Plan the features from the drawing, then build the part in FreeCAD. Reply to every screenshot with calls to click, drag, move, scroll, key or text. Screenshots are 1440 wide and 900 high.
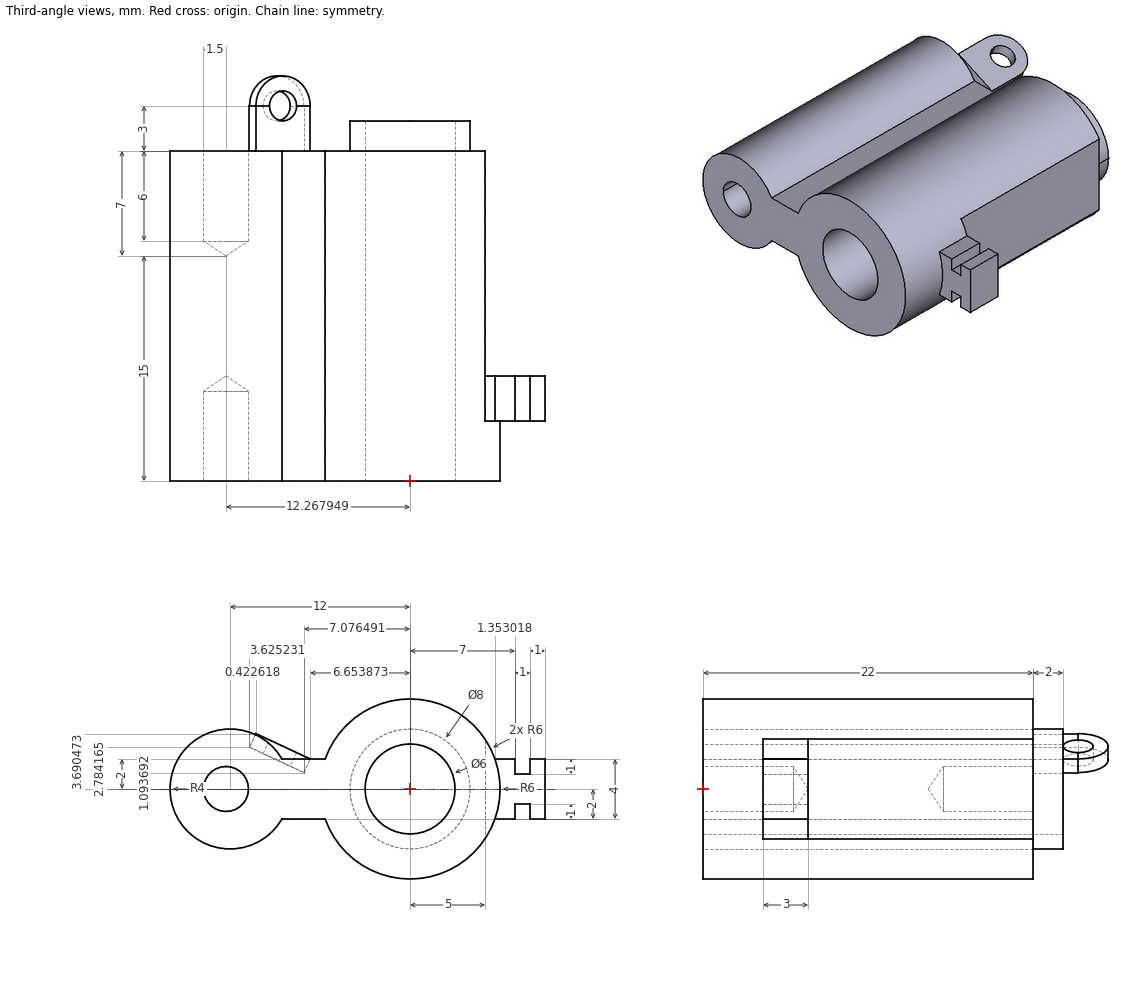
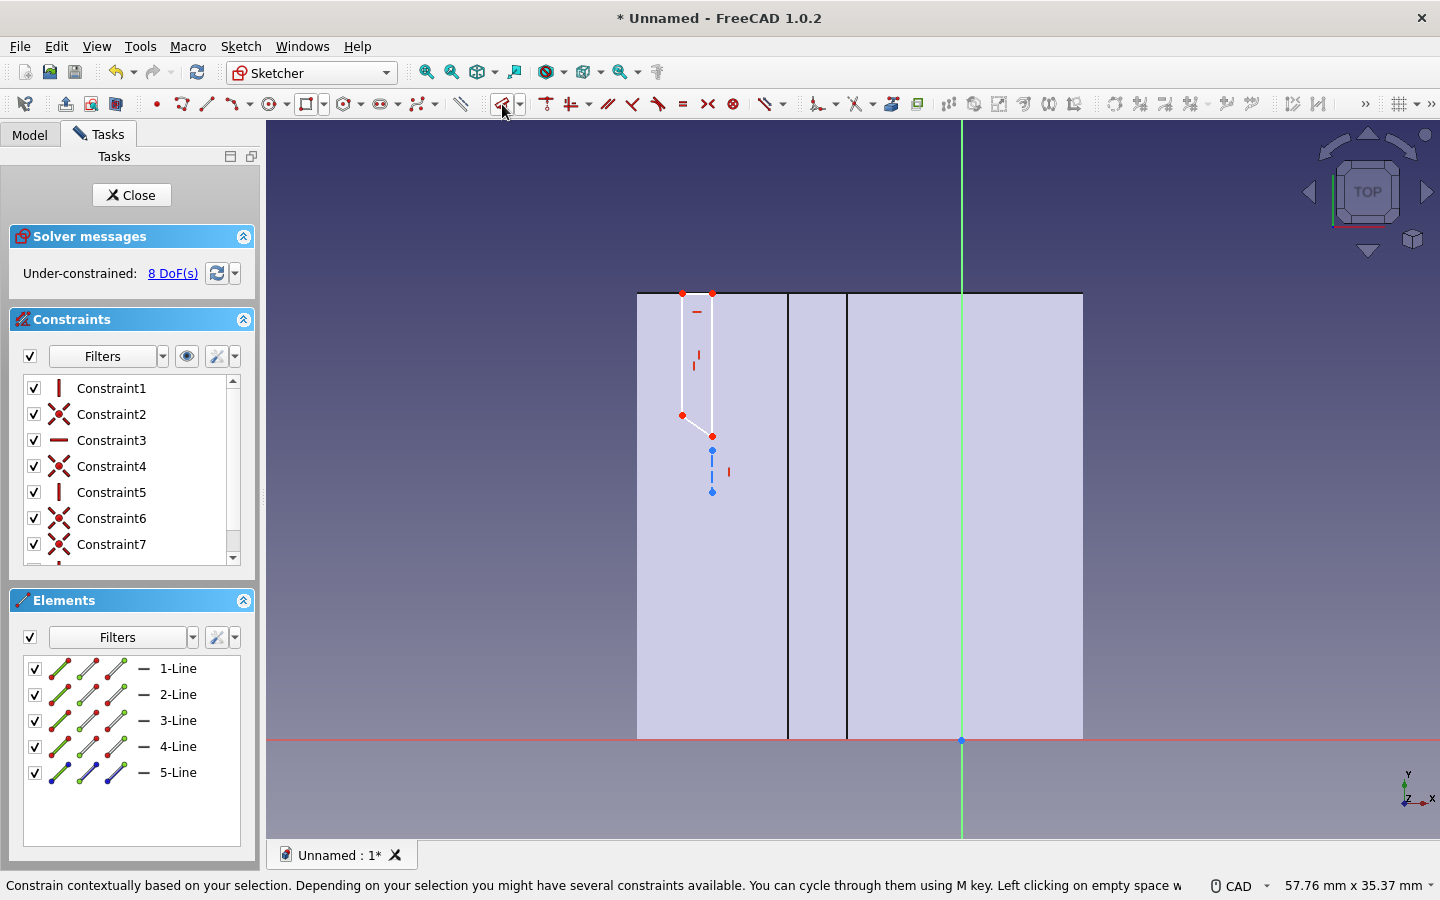
click(712, 394)
click(746, 366)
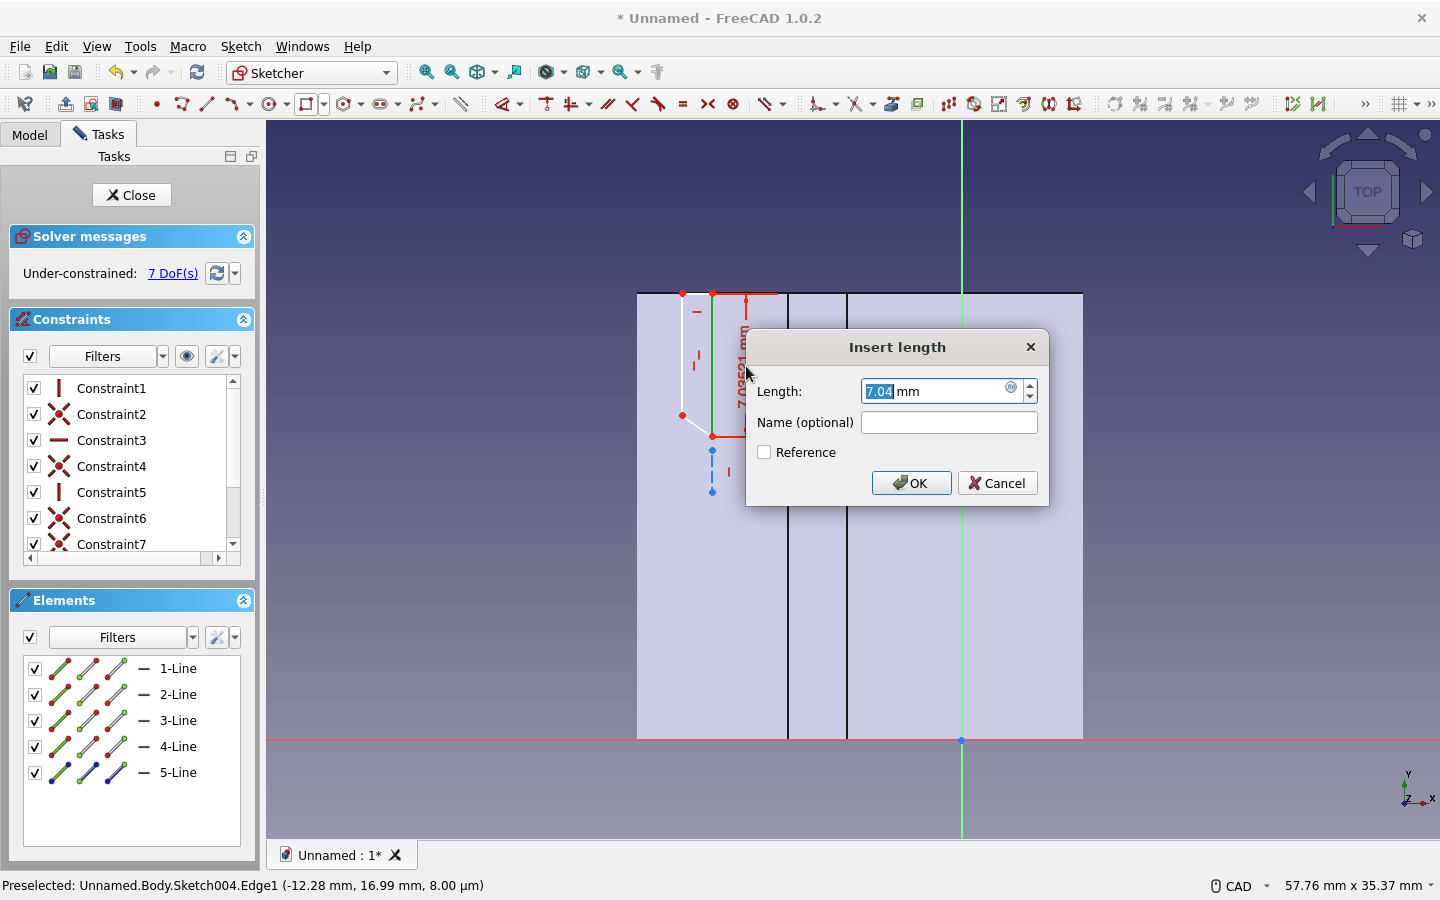
text(7)
key(Return)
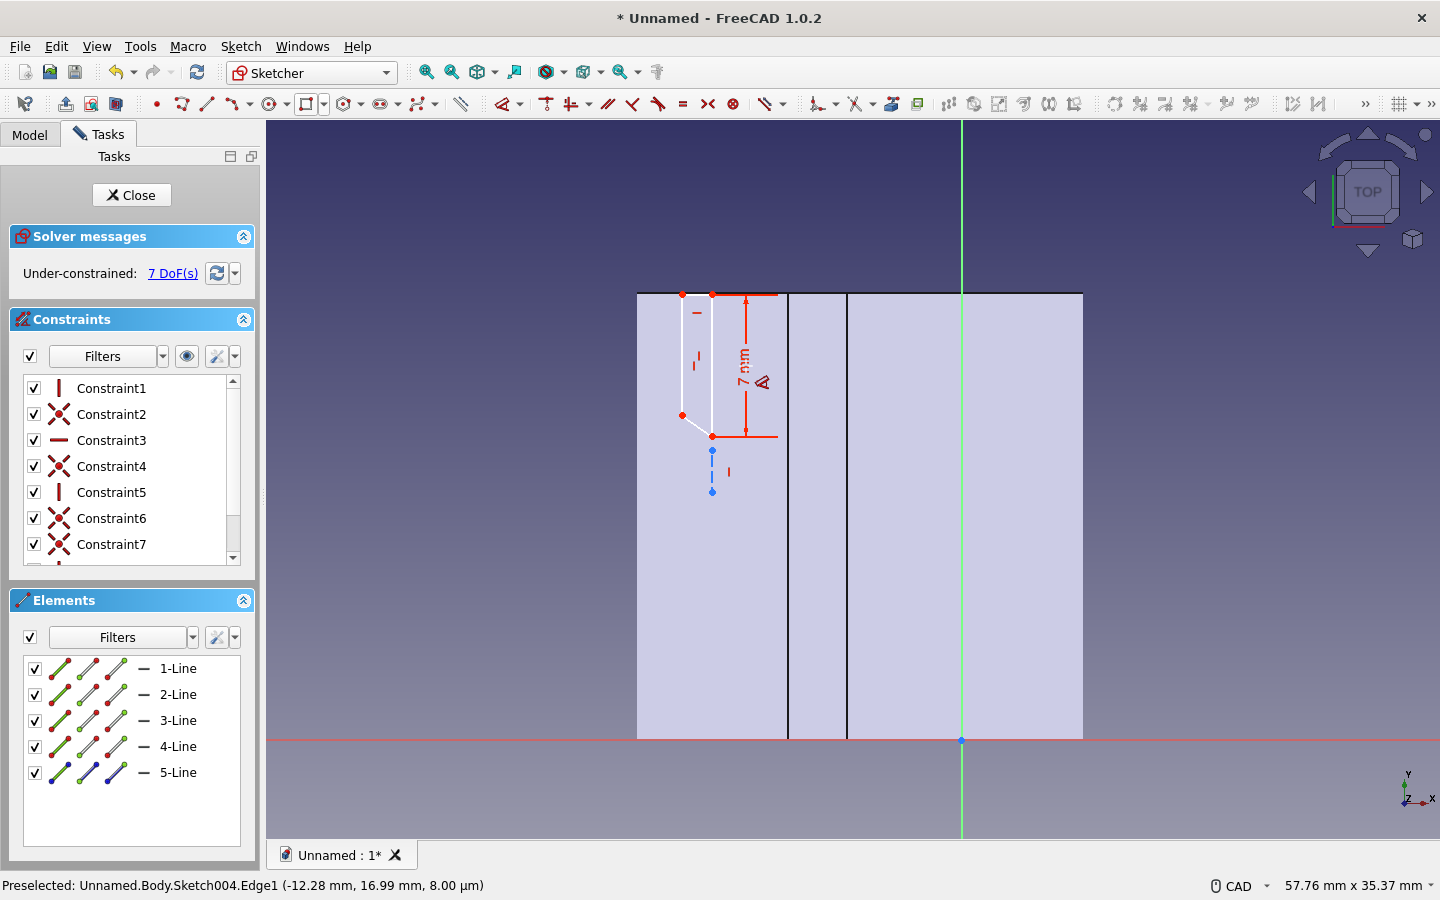
click(682, 331)
click(648, 355)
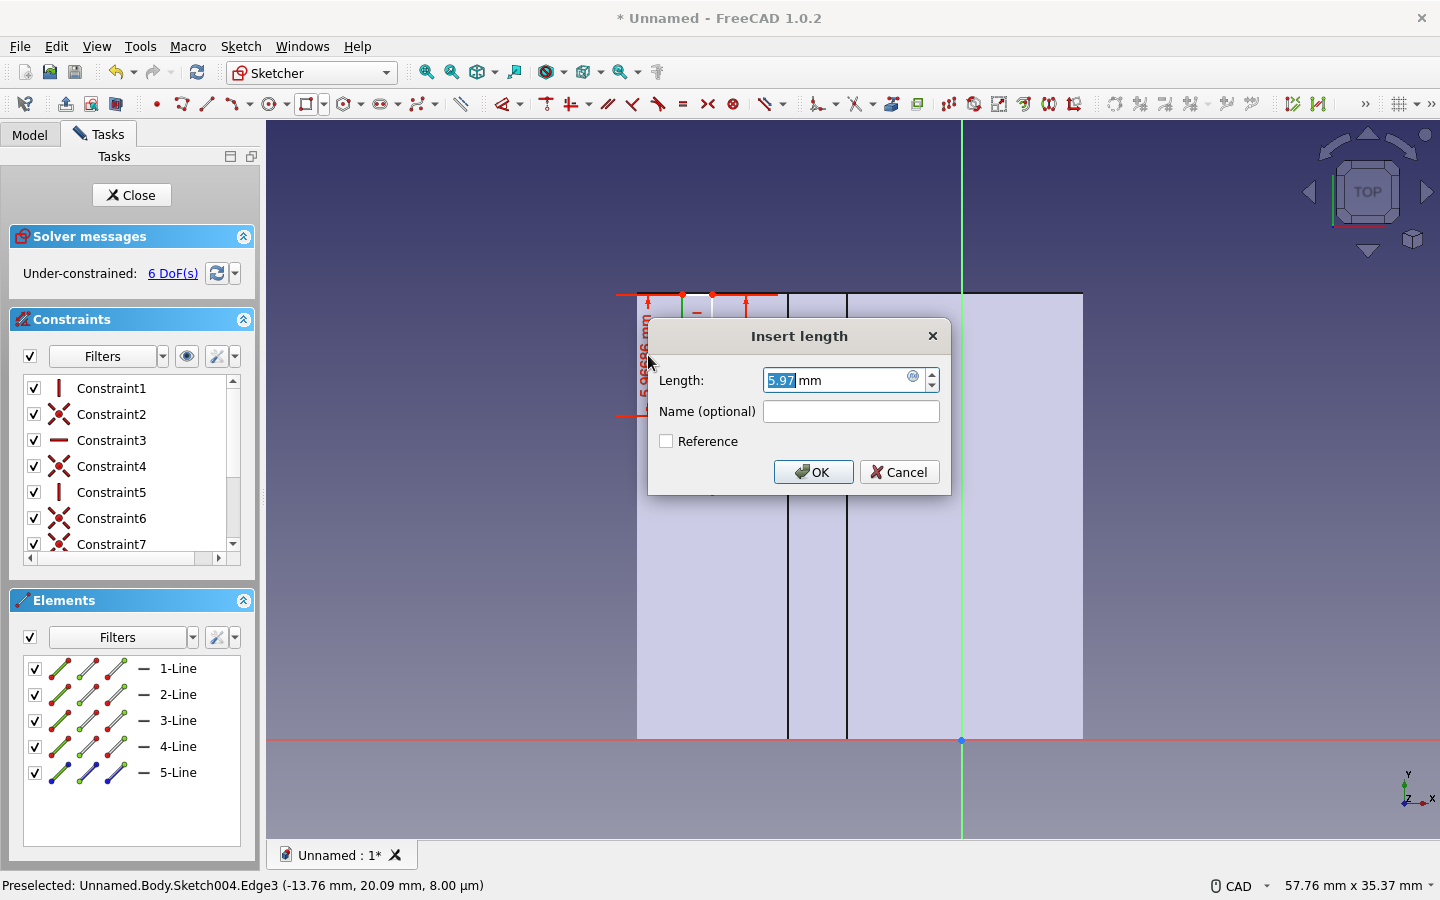
text(6)
key(Return)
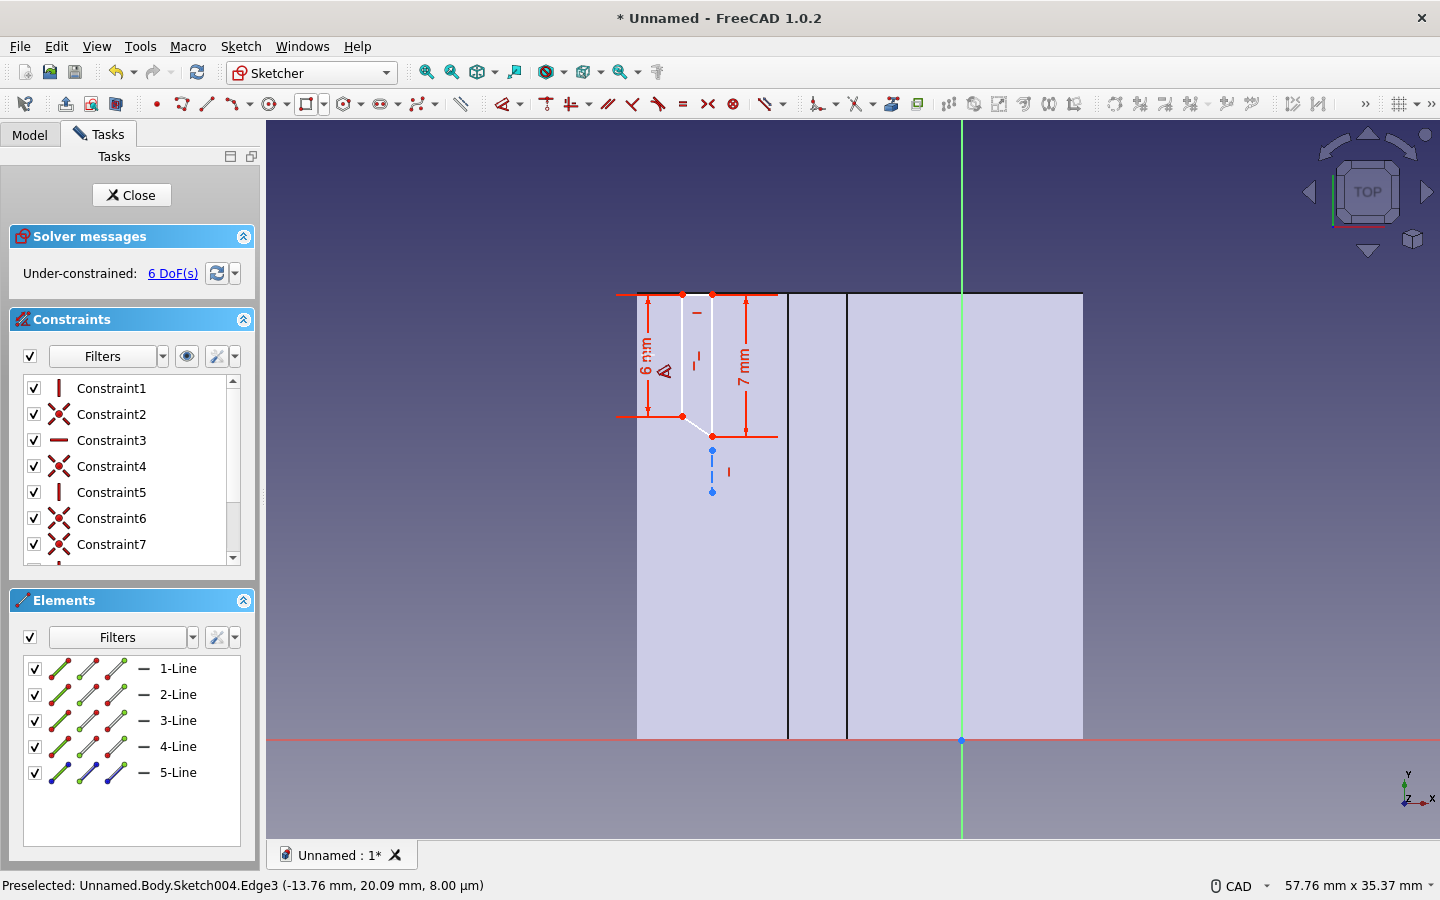
scroll(700, 295, up, 2)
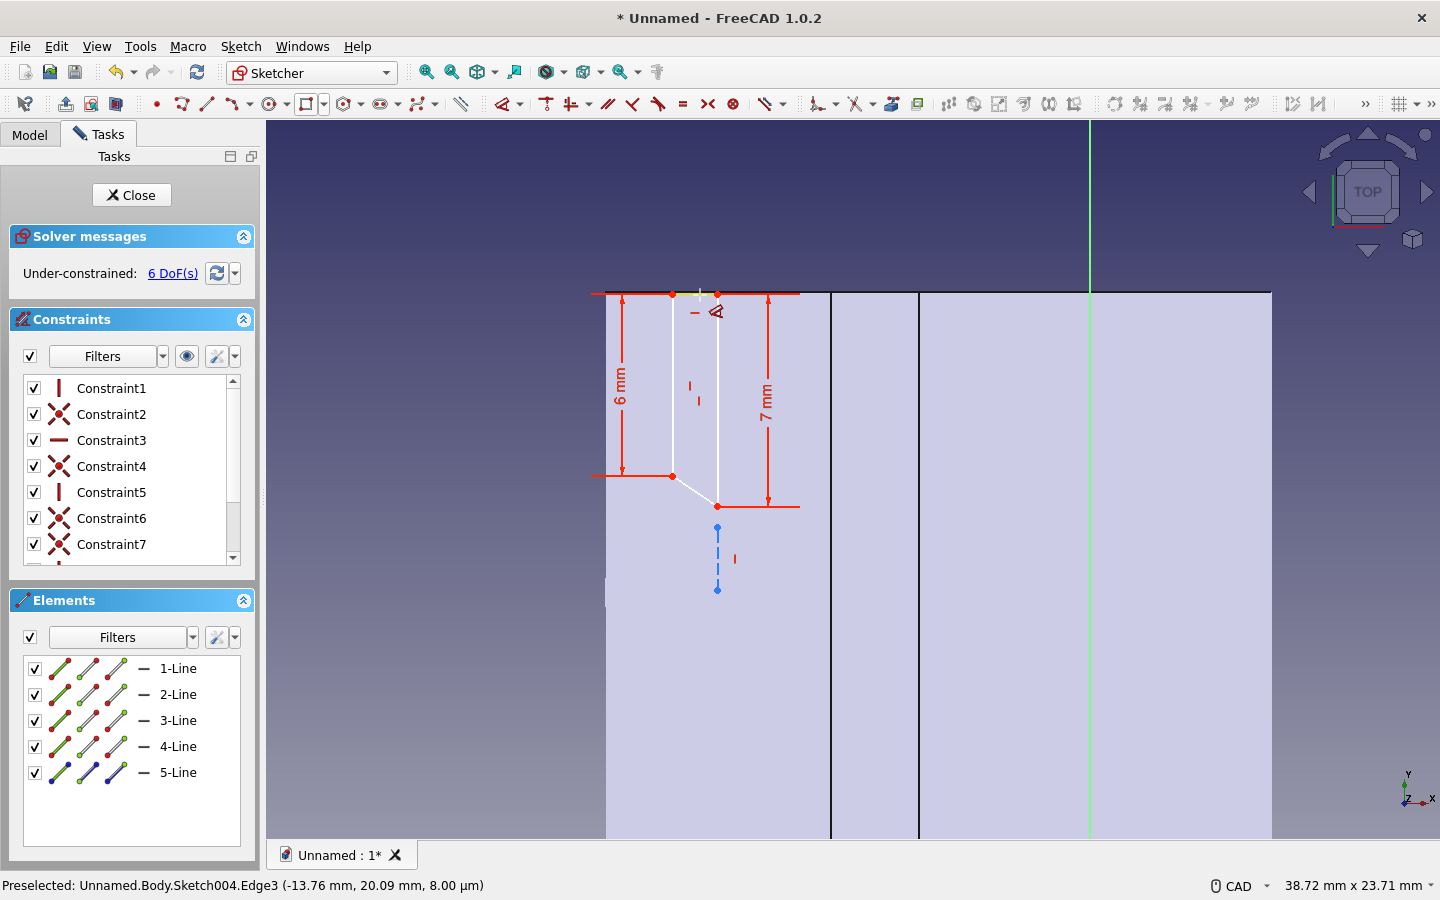
click(700, 294)
click(695, 260)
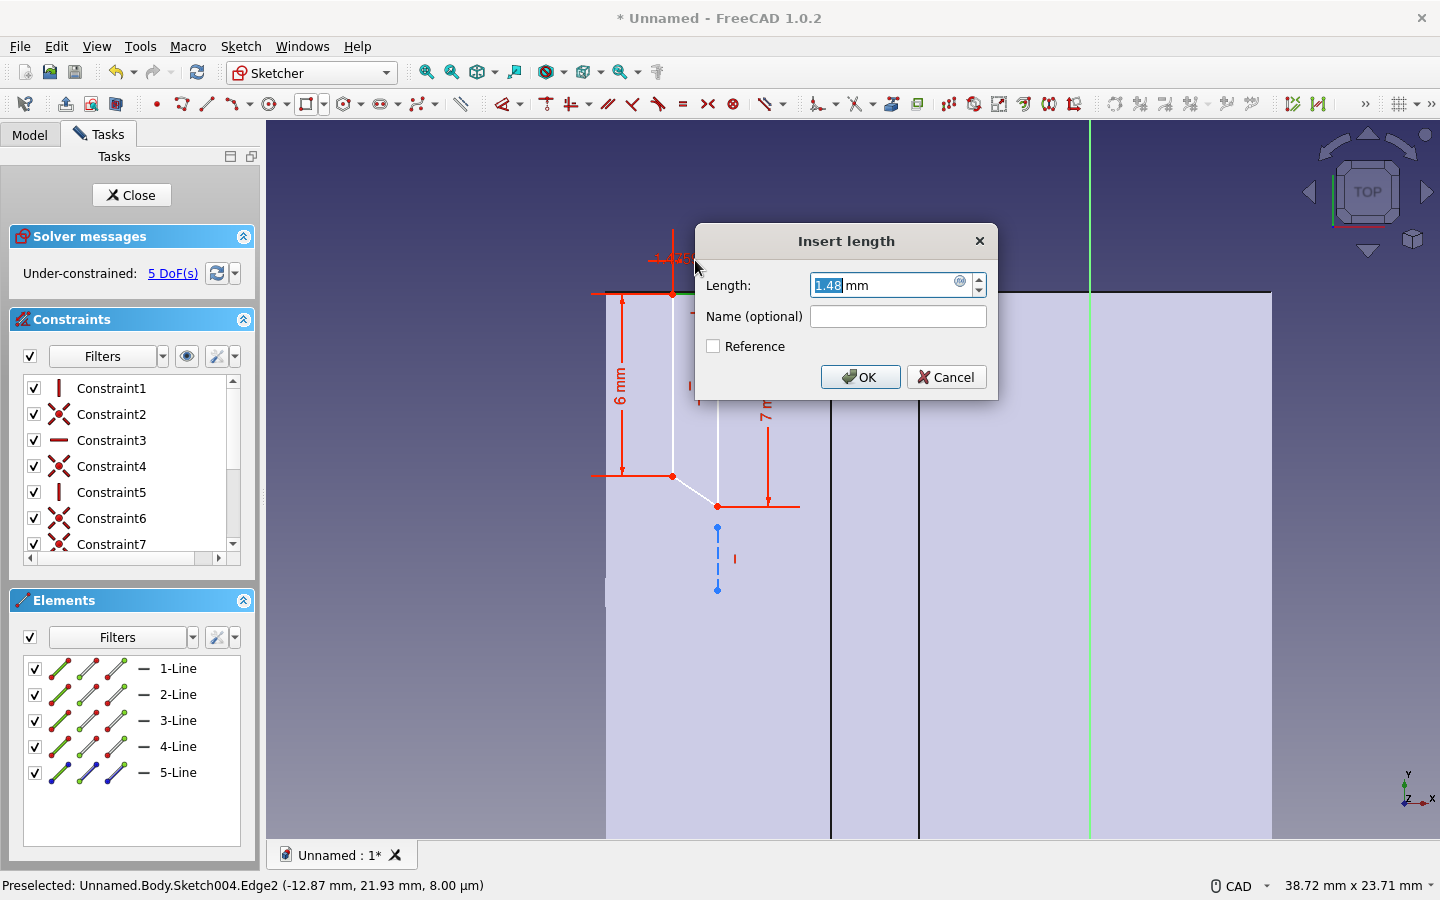
text(1.5)
key(Return)